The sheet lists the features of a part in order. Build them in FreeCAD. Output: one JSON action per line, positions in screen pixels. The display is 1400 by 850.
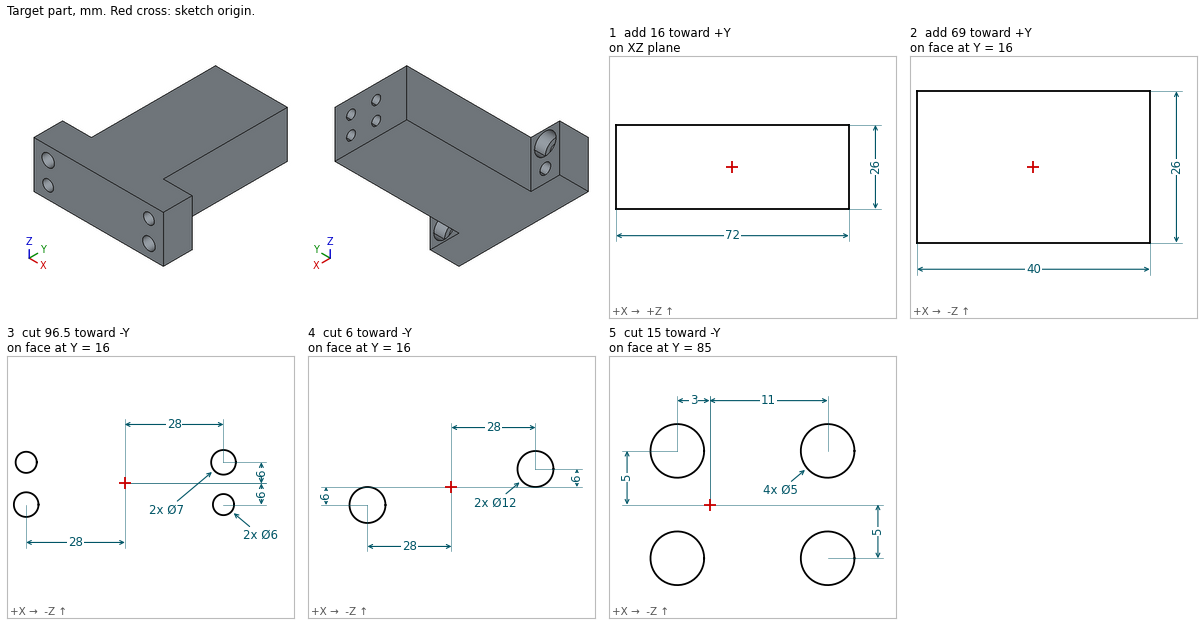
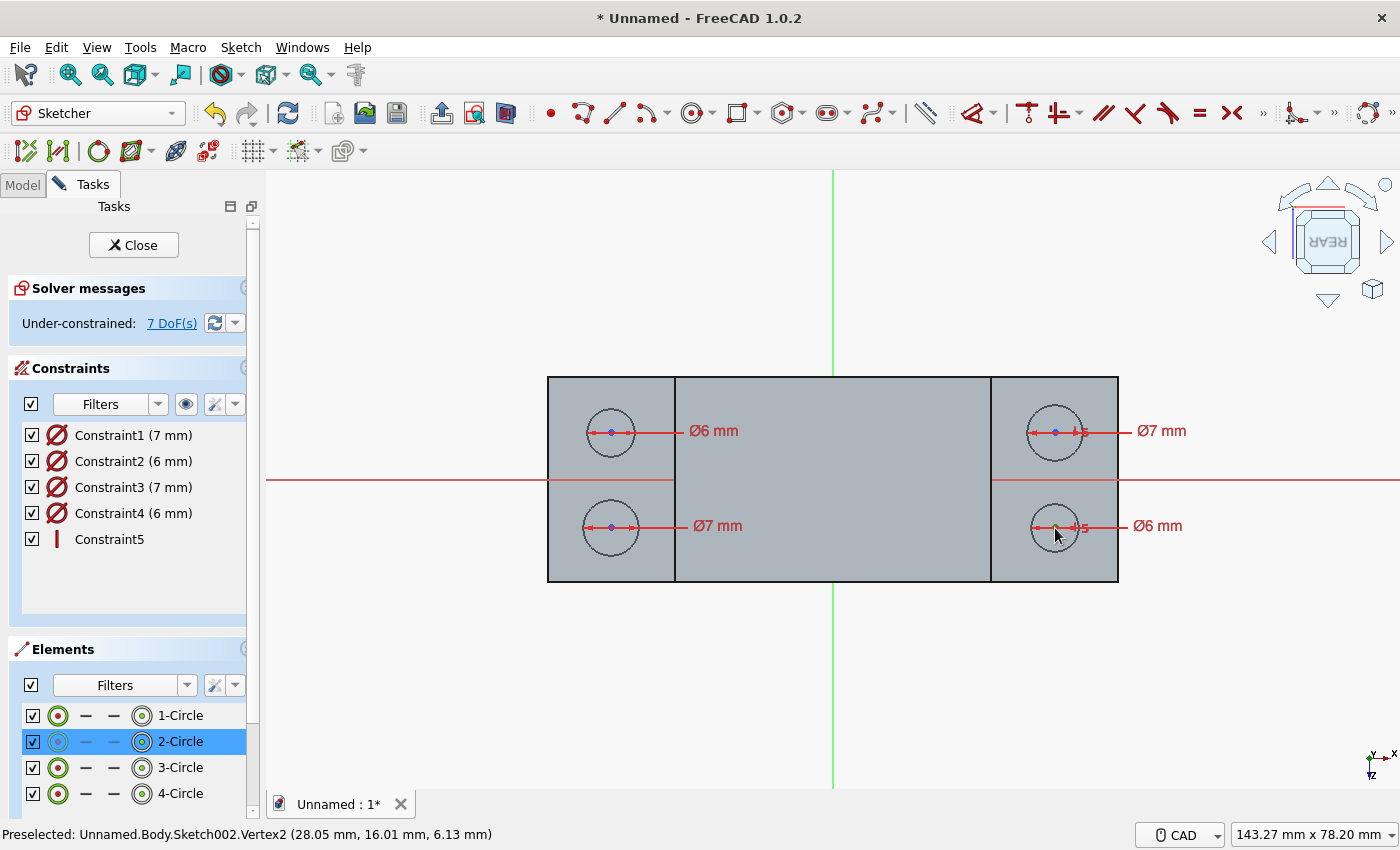
{"action": "left_click", "coordinate": [611, 528]}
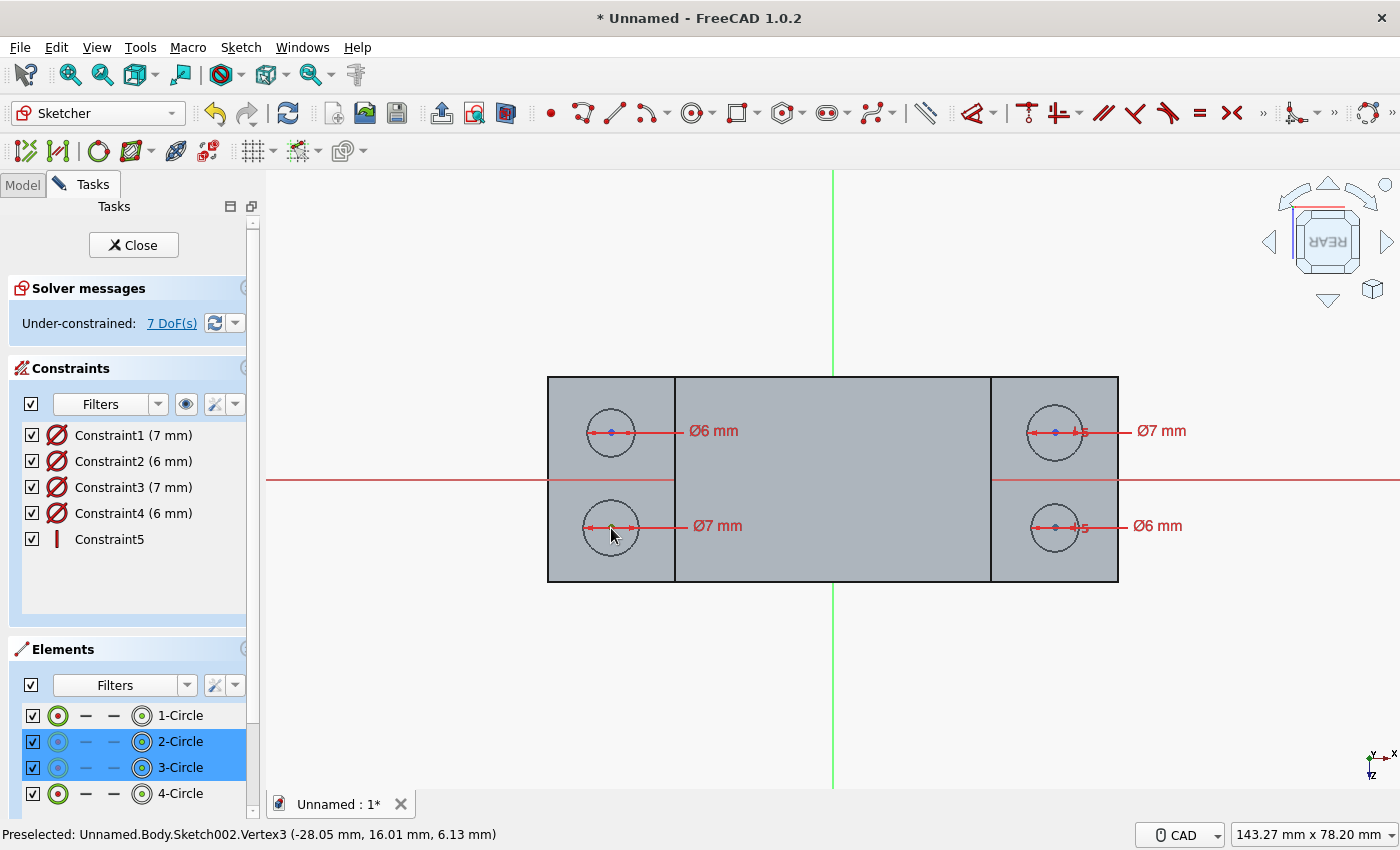
{"action": "left_click", "coordinate": [1082, 114]}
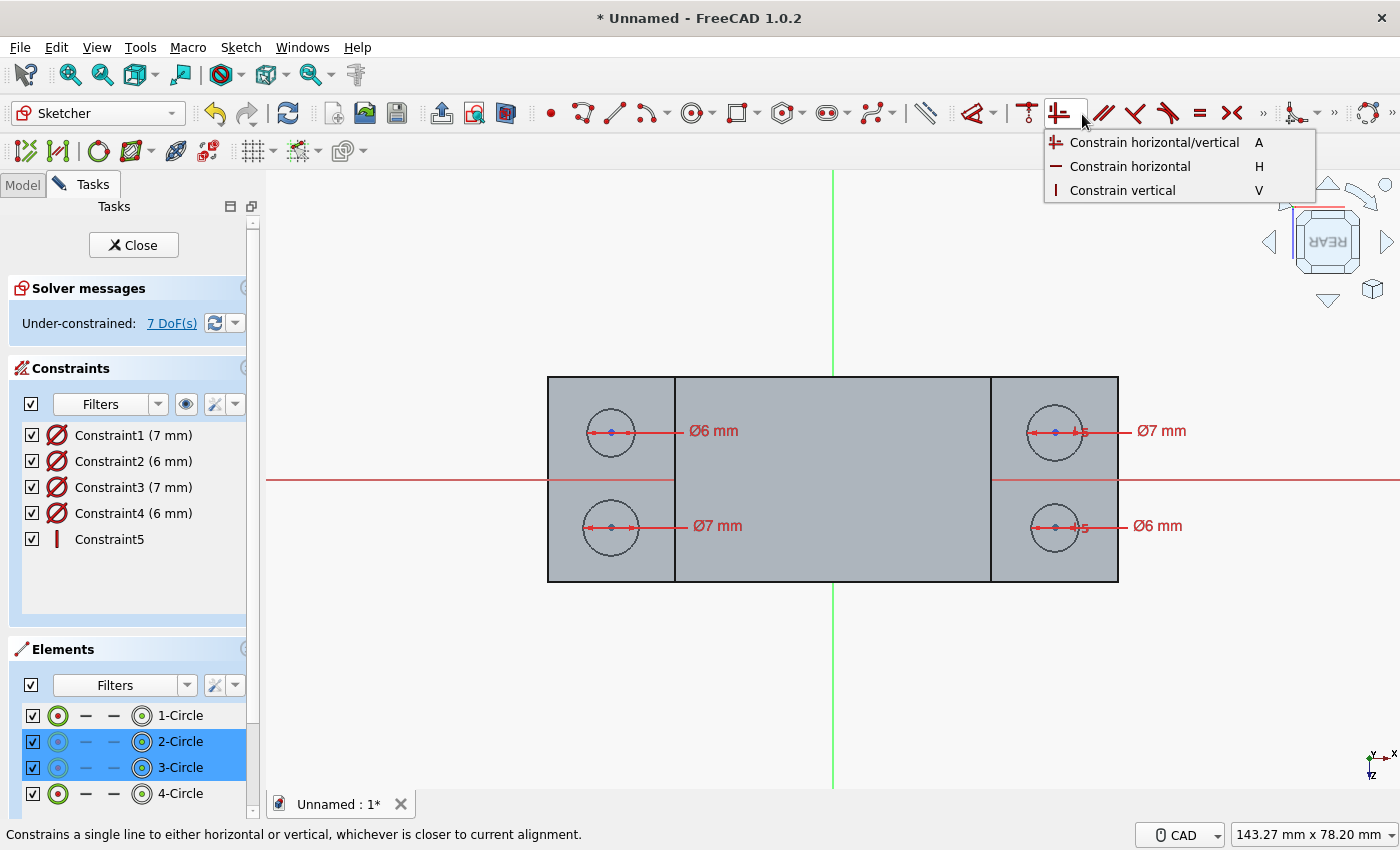
{"action": "left_click", "coordinate": [1180, 166]}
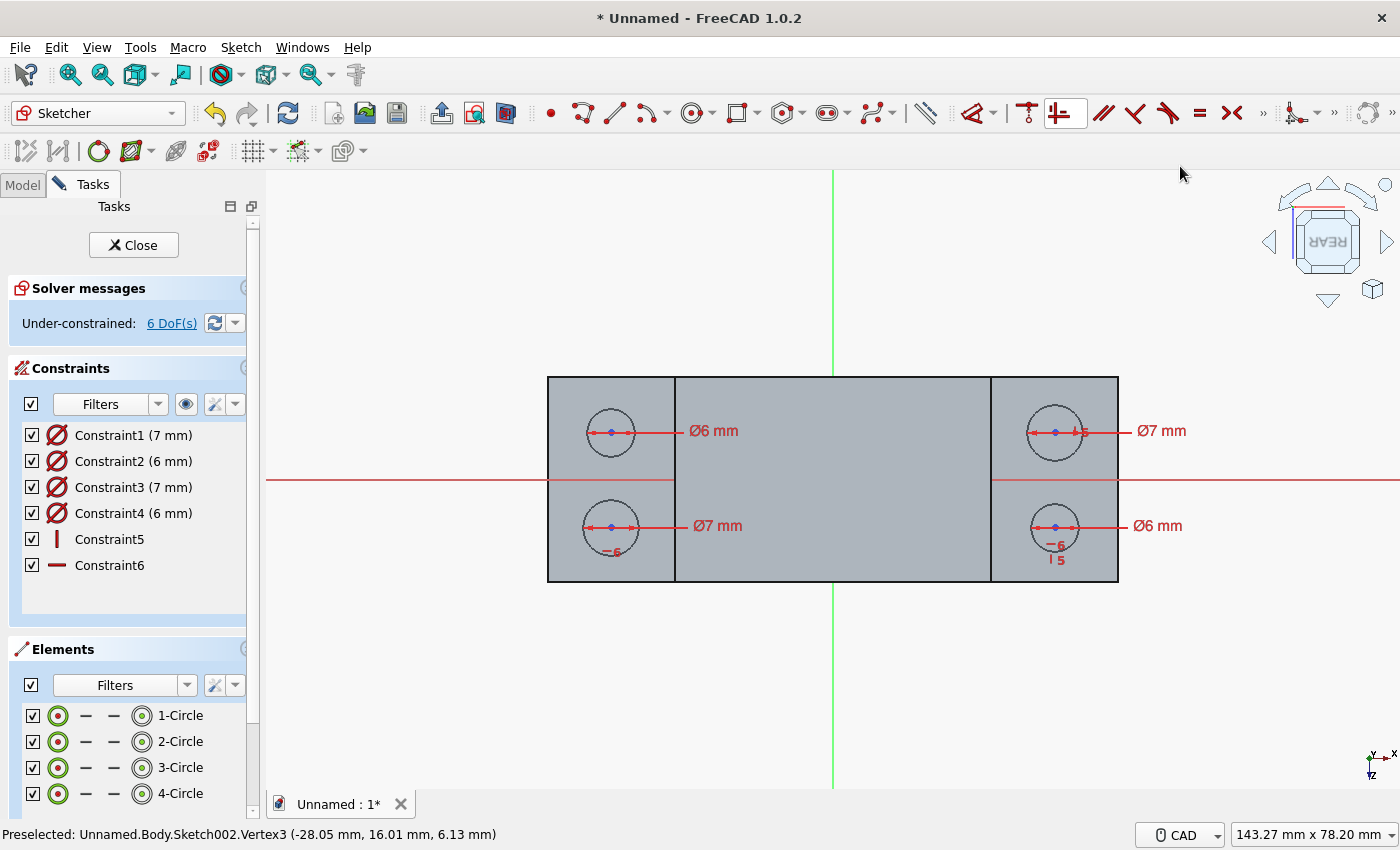
{"action": "left_click", "coordinate": [611, 528]}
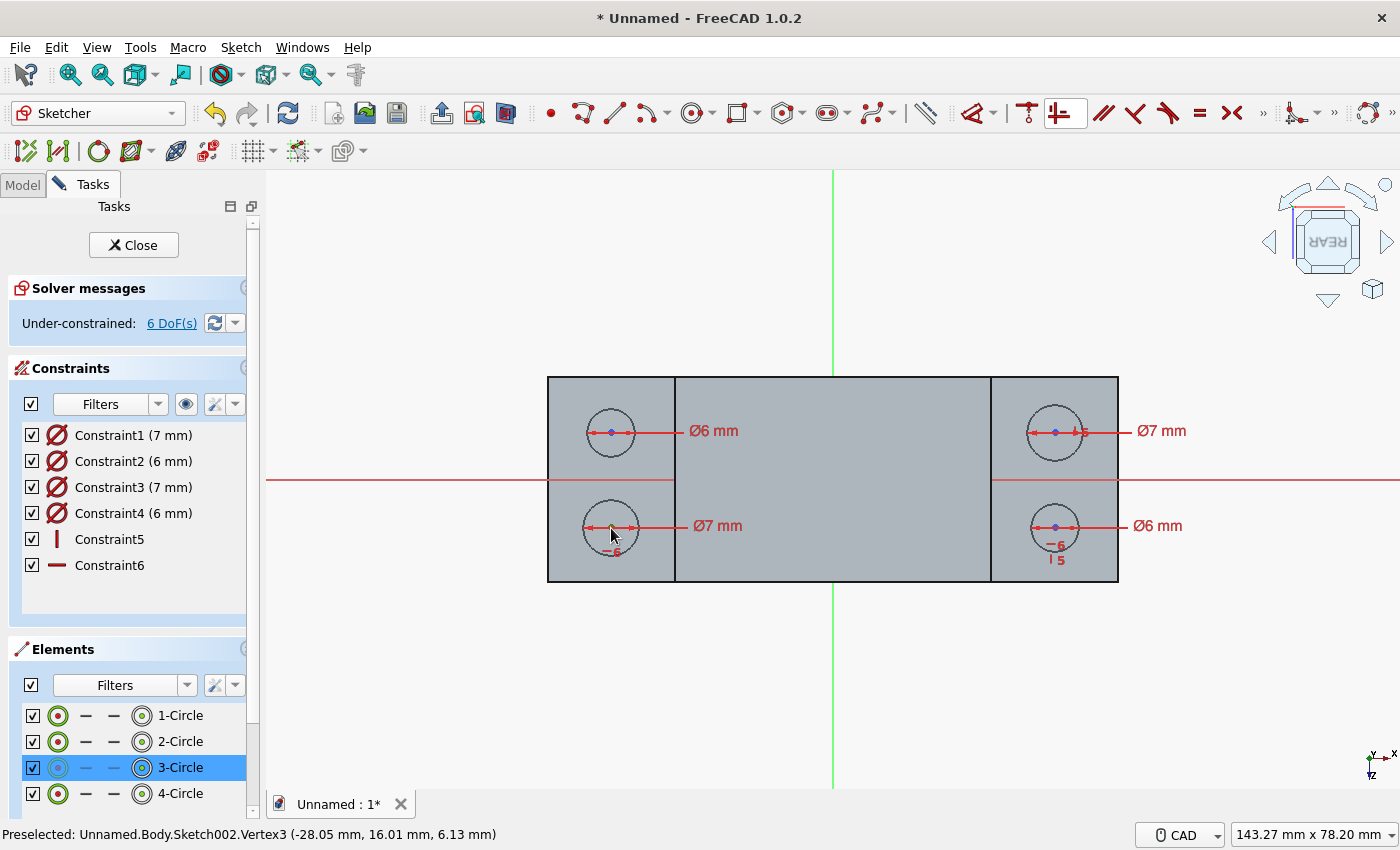
{"action": "left_click", "coordinate": [611, 433]}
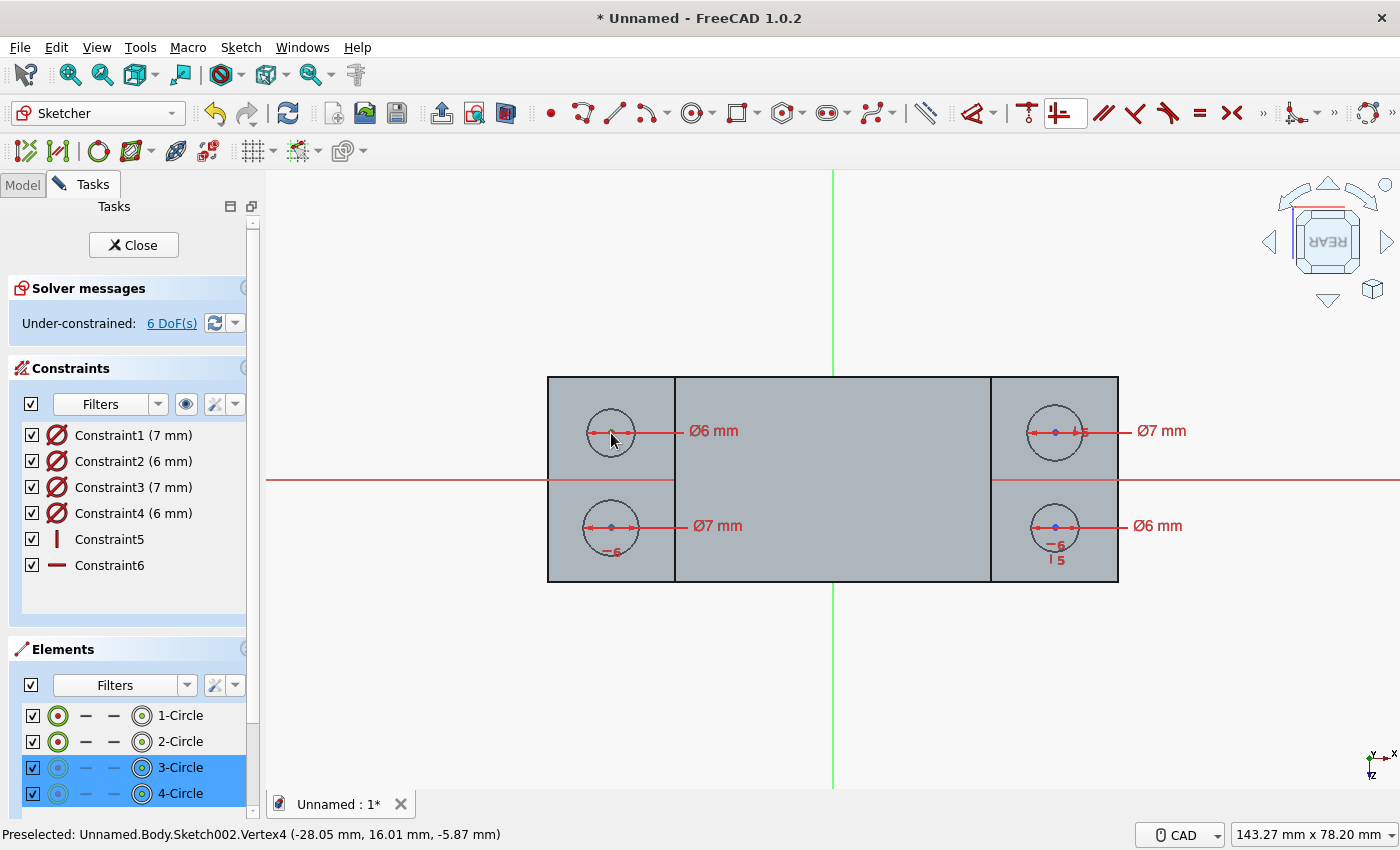
{"action": "key", "text": "v"}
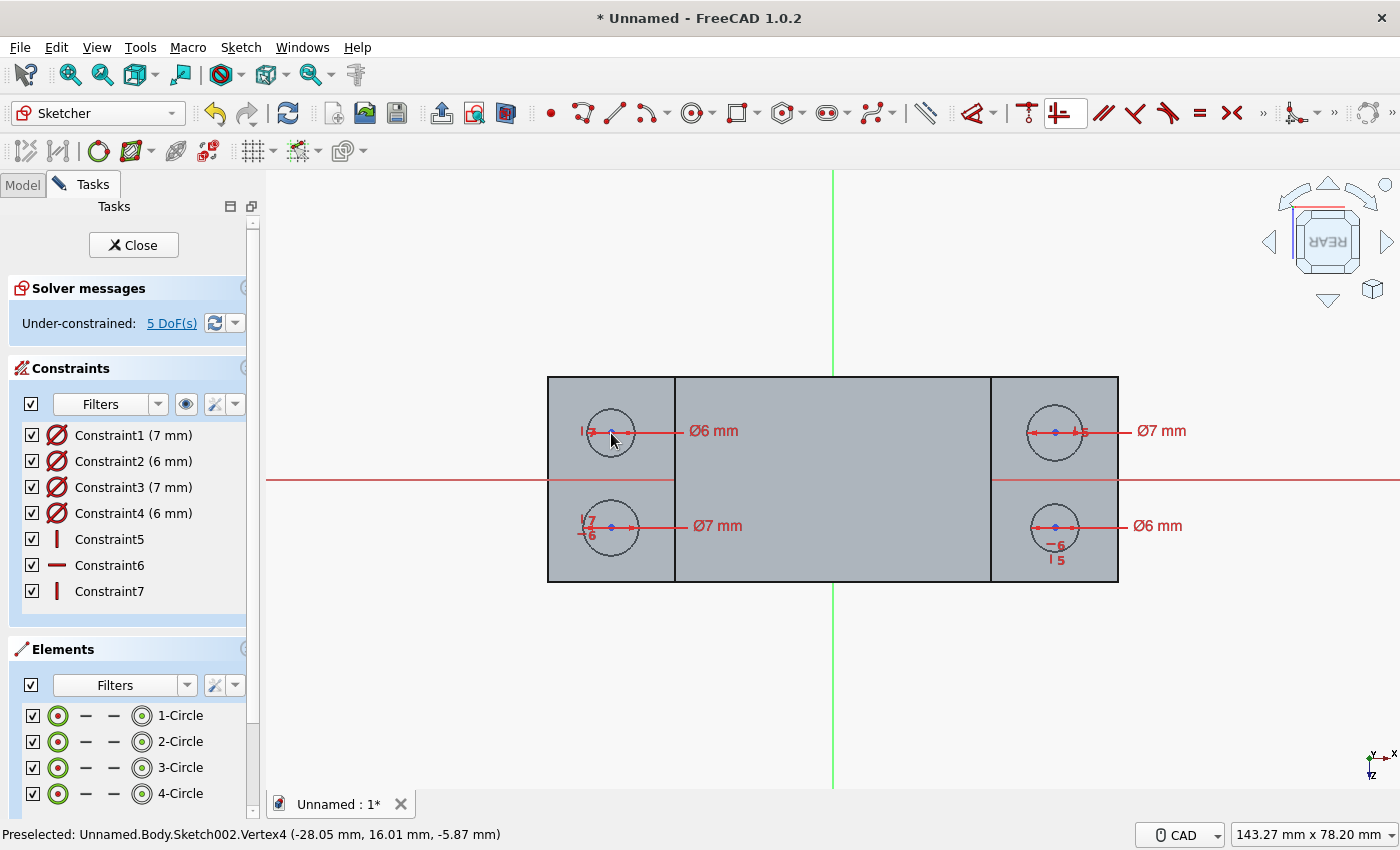
{"action": "left_click", "coordinate": [1055, 433]}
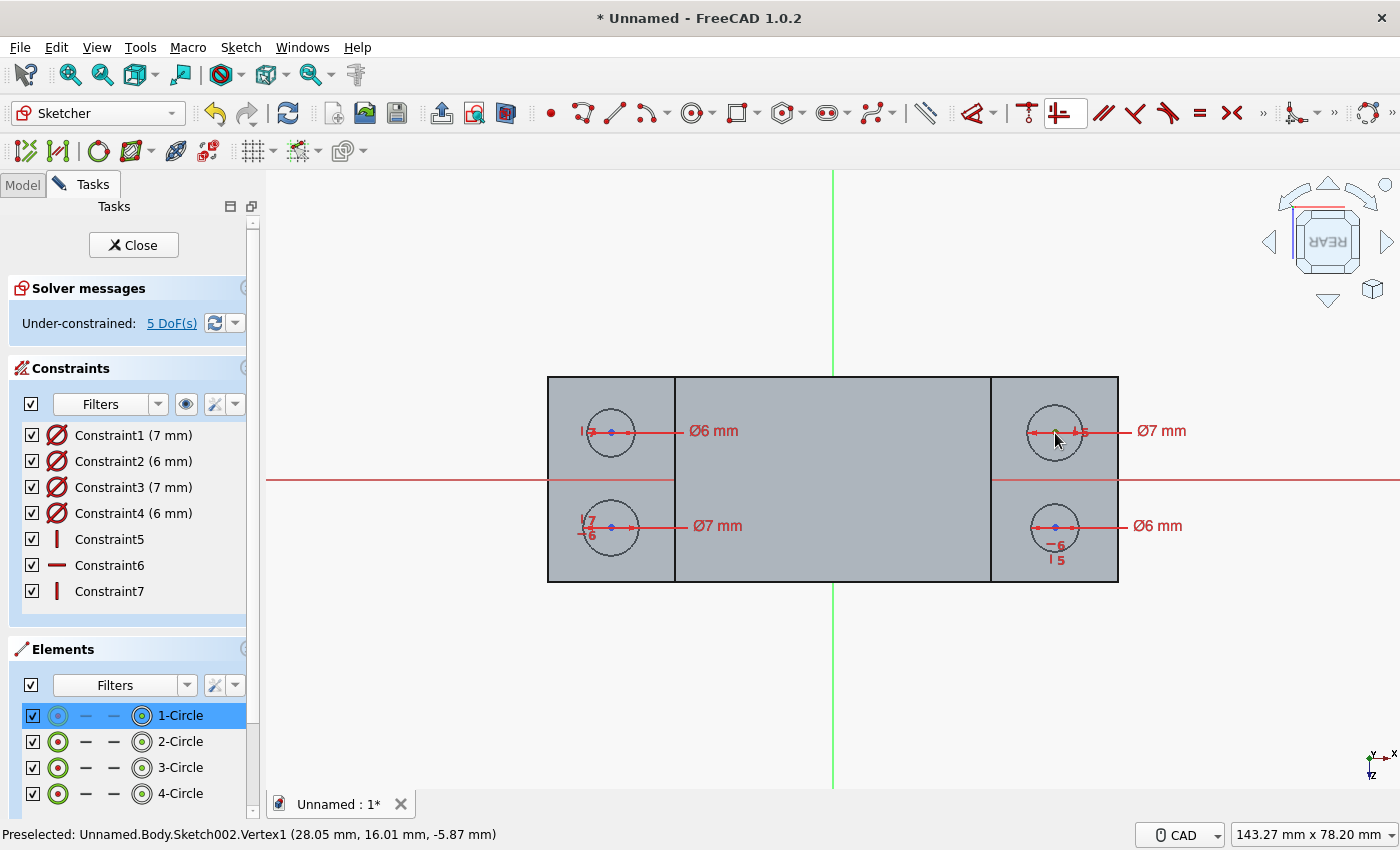
{"action": "left_click", "coordinate": [611, 433]}